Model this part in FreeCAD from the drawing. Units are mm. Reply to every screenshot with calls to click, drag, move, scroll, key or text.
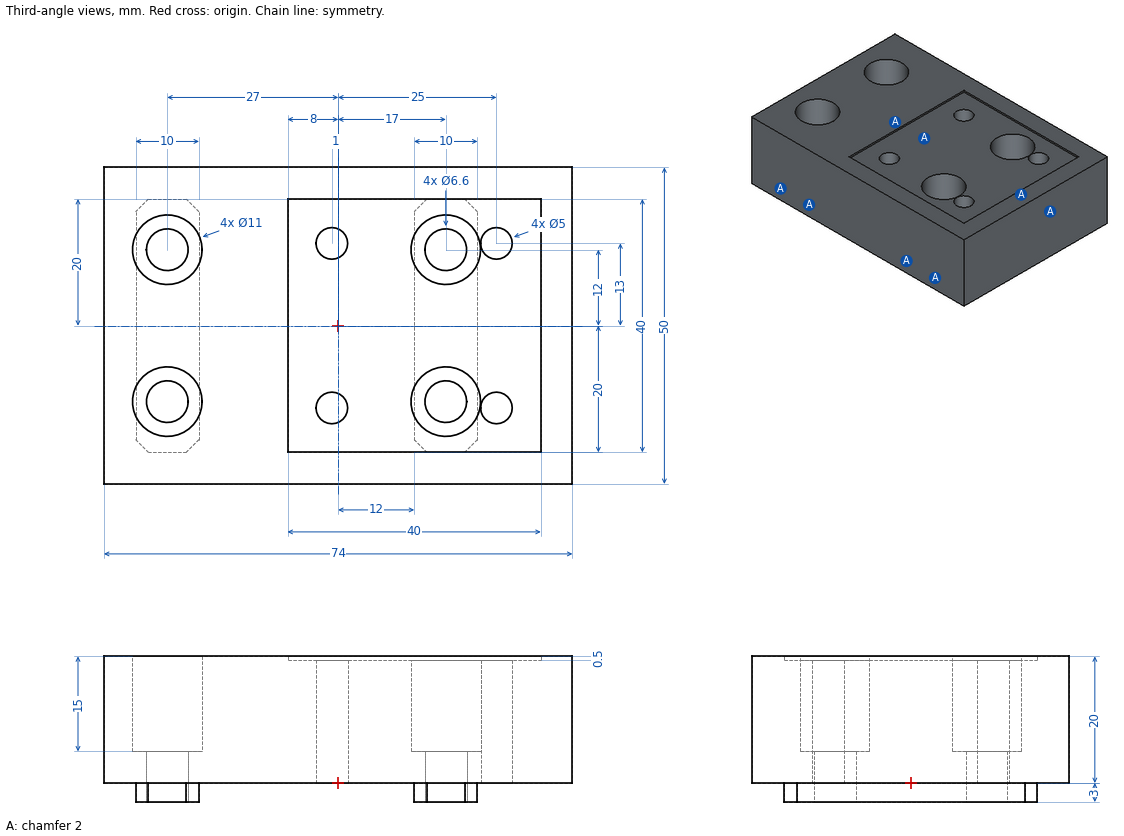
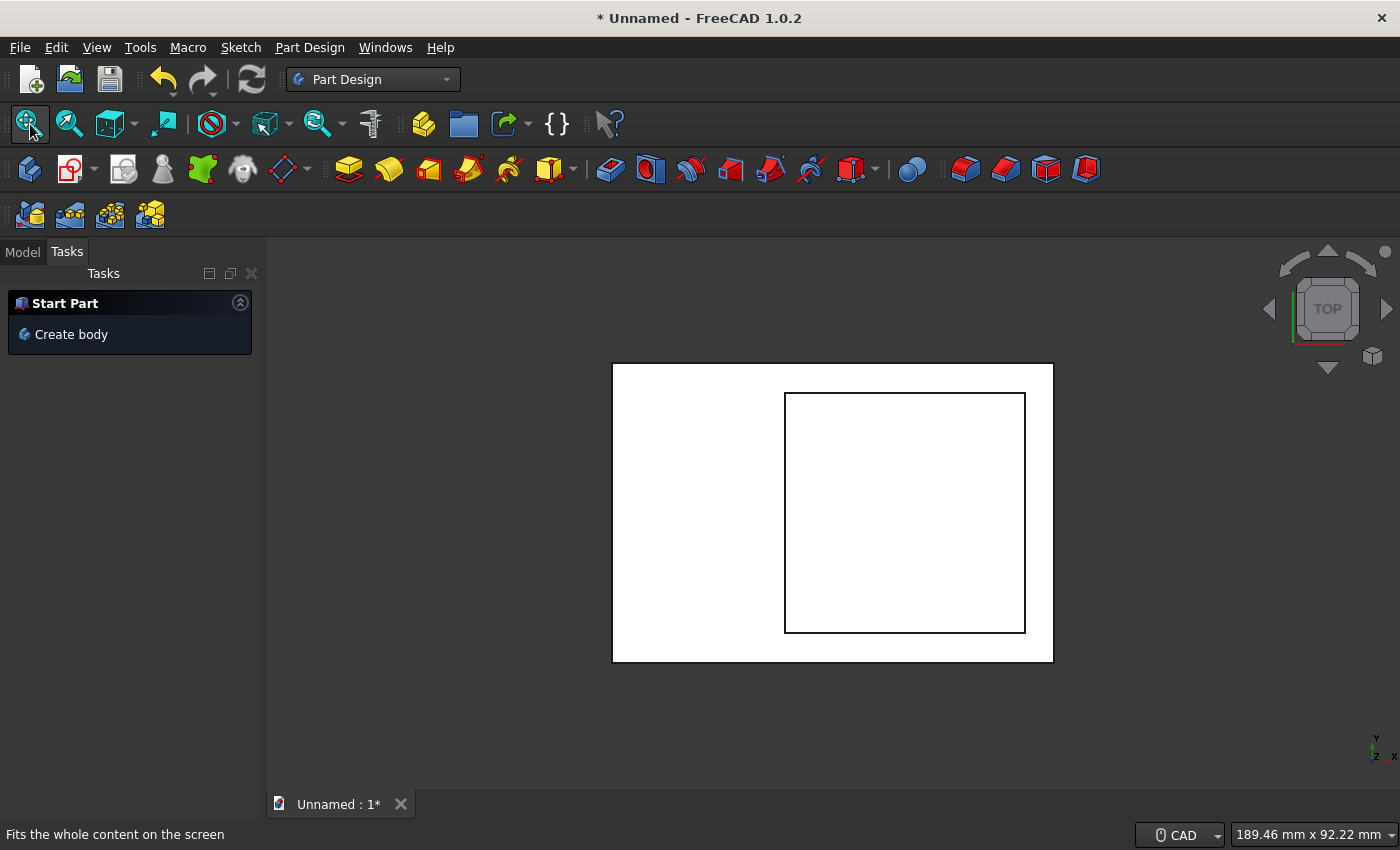
scroll(965, 392, up, 5)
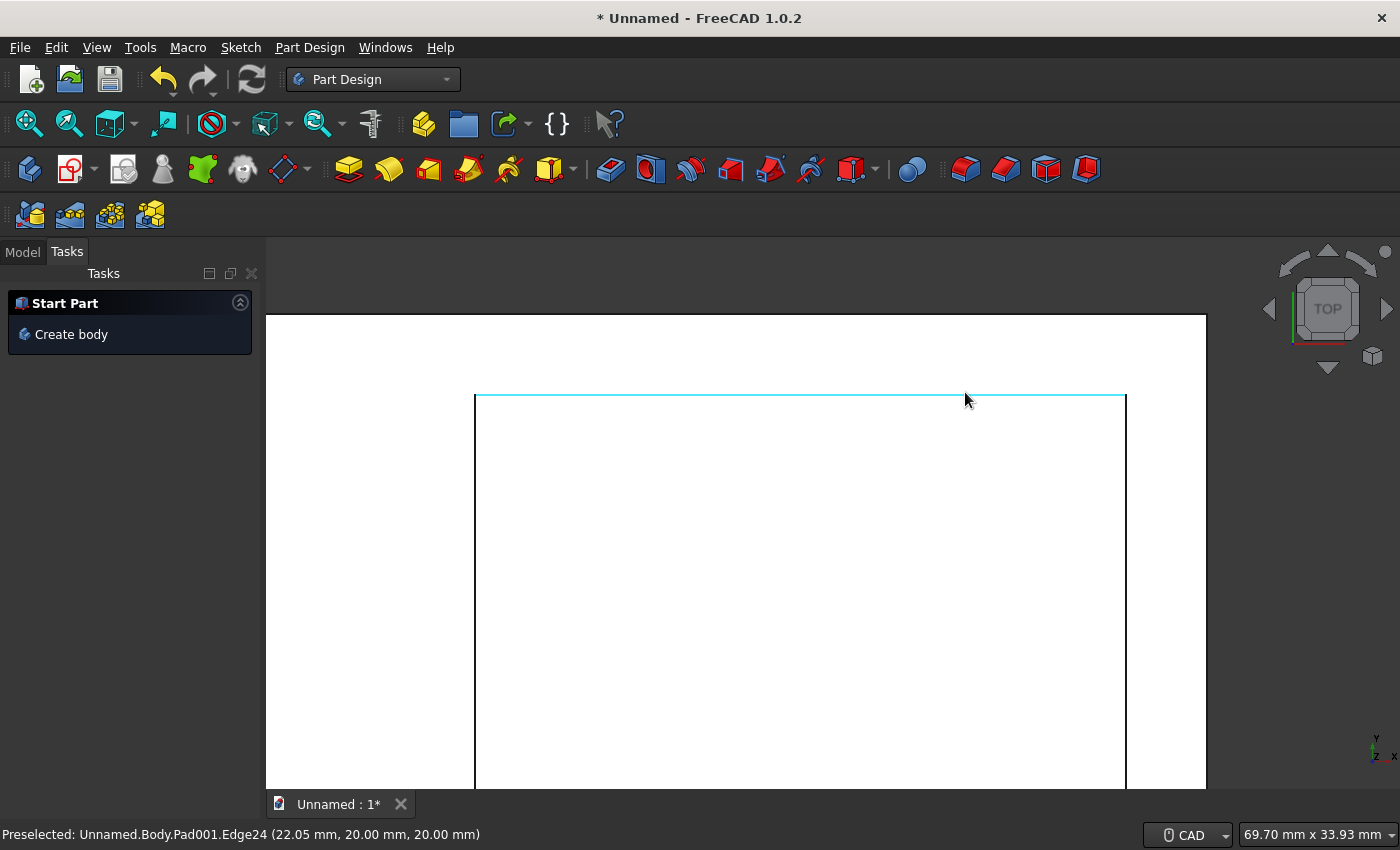
click(30, 124)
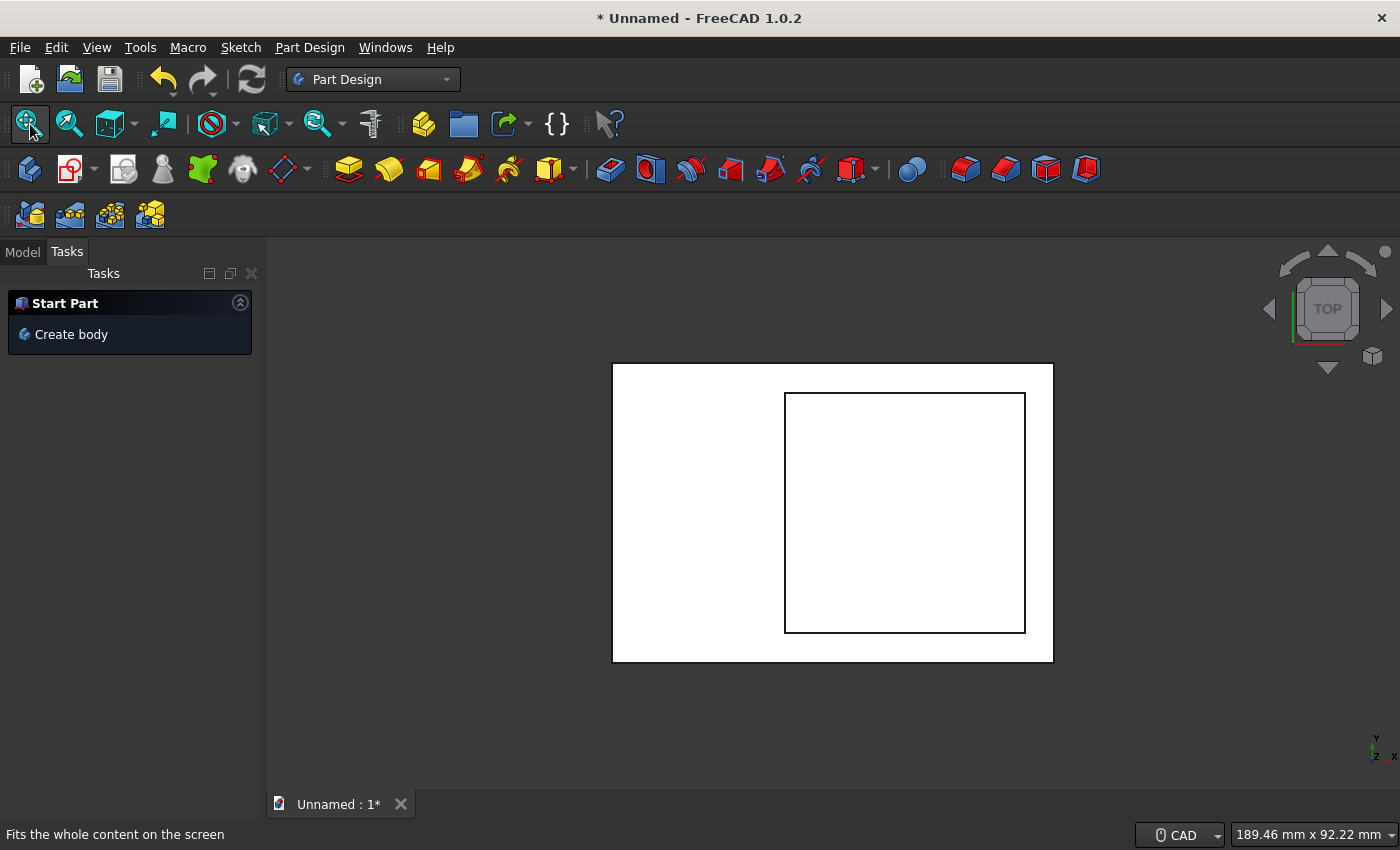
key(1)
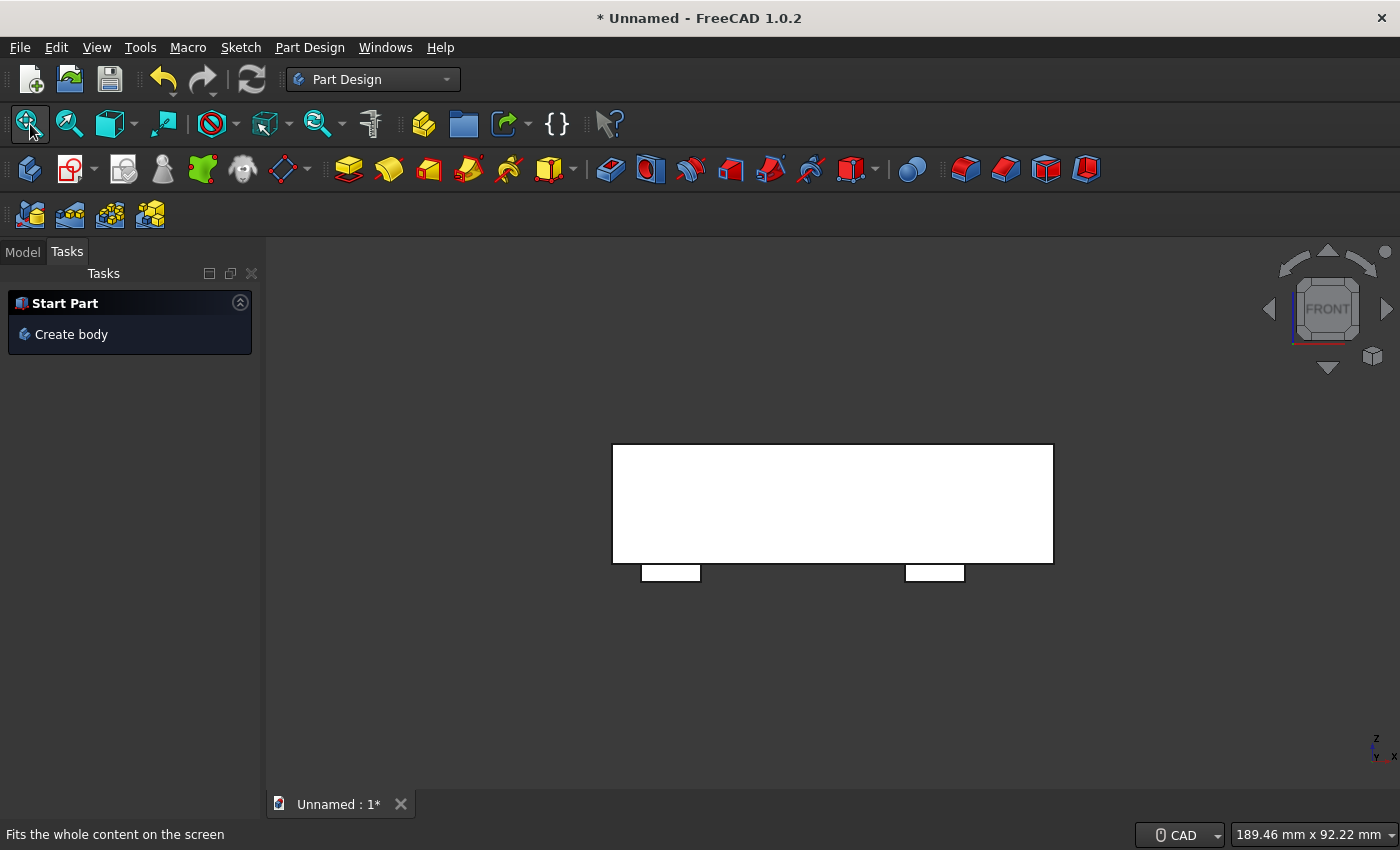
click(30, 124)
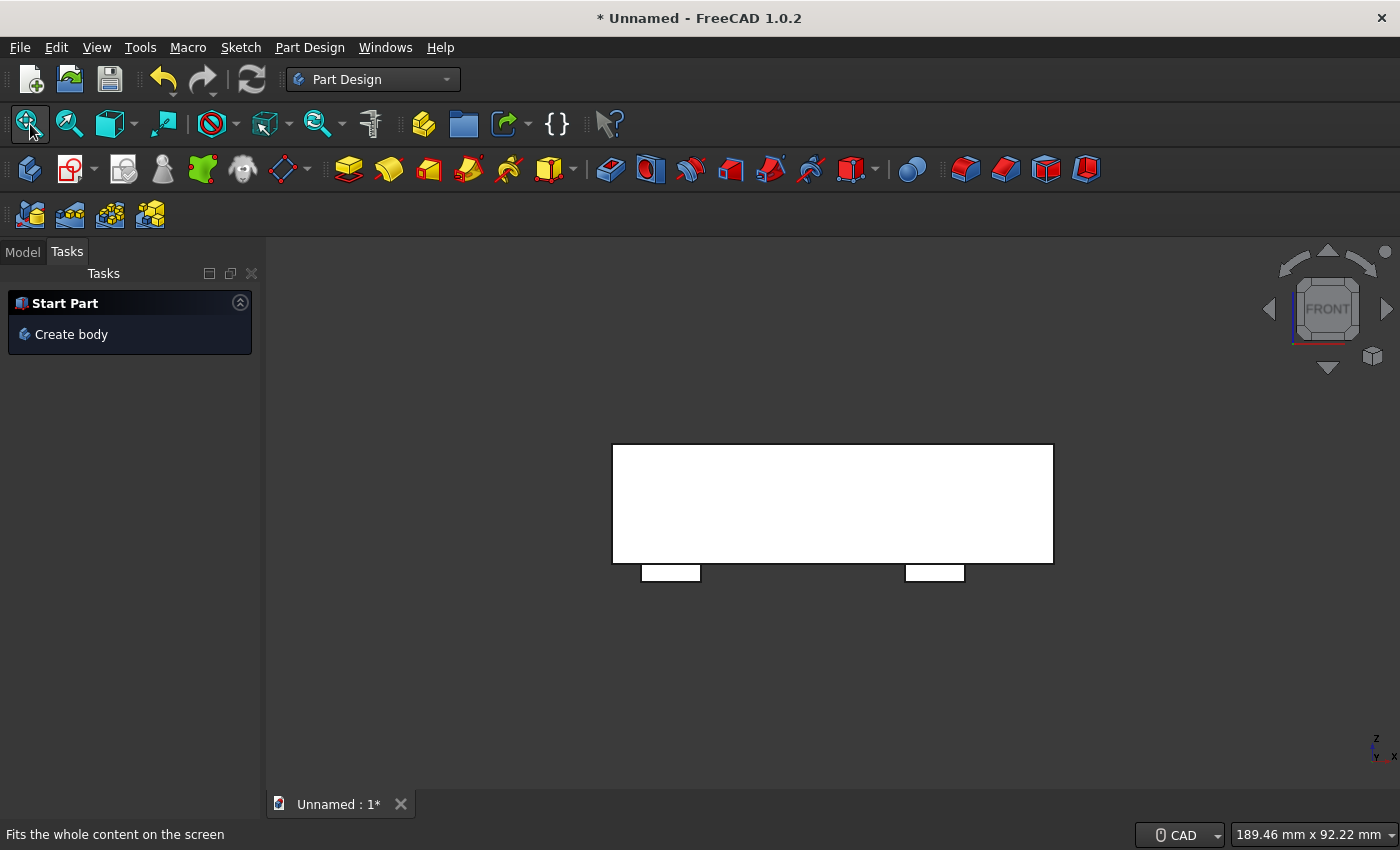
click(965, 572)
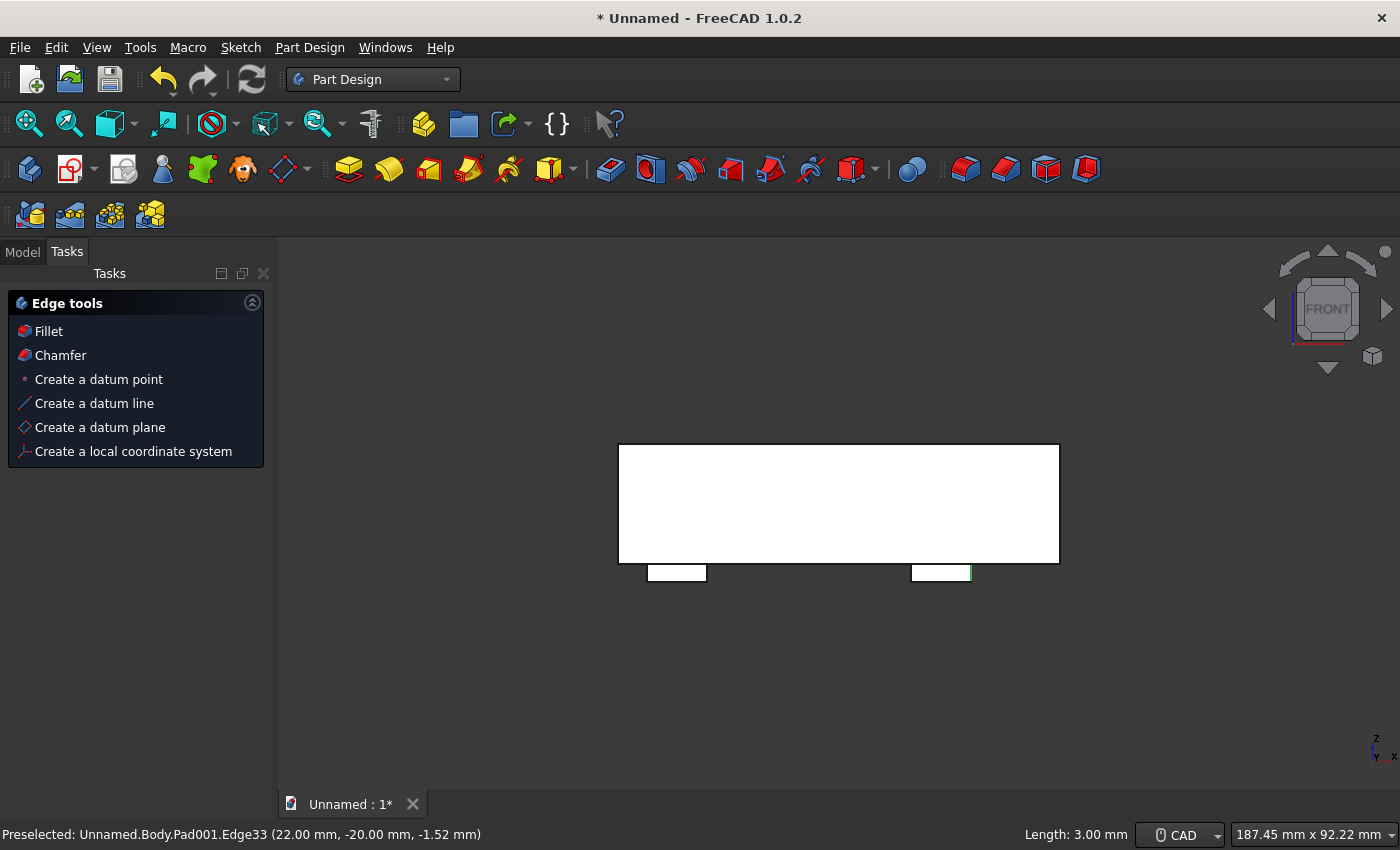
click(911, 572, ctrl)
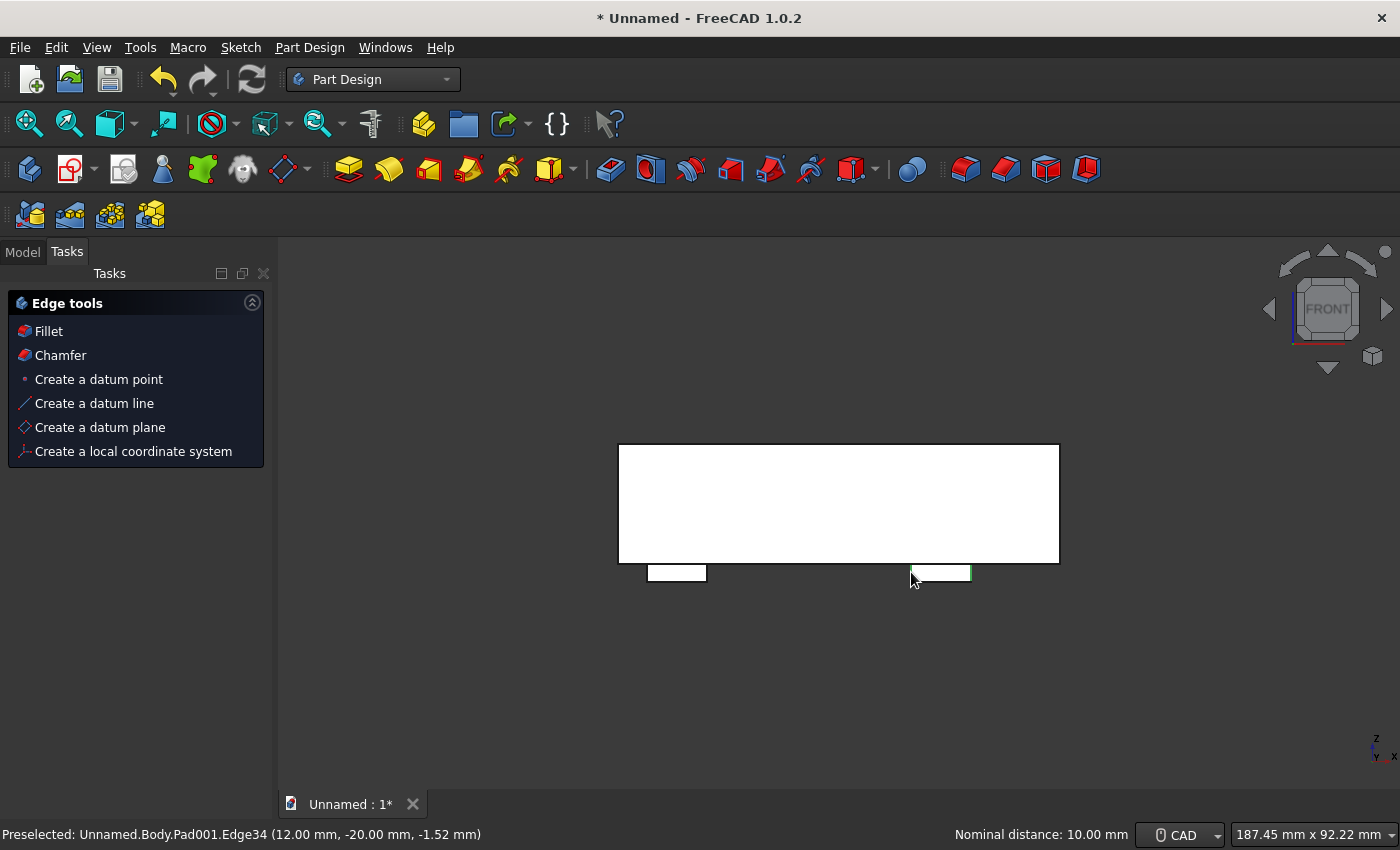
click(707, 572, ctrl)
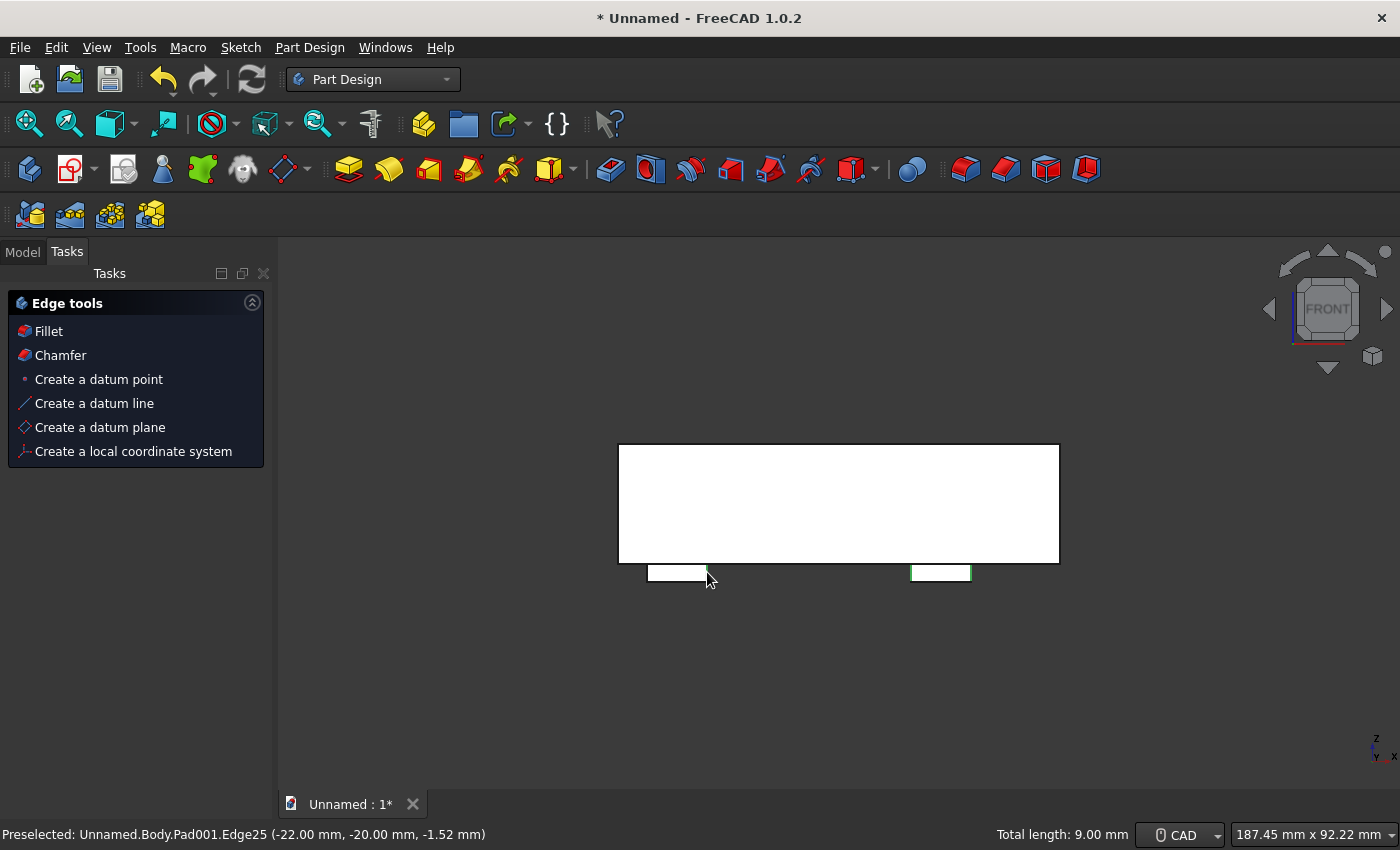
click(647, 572, ctrl)